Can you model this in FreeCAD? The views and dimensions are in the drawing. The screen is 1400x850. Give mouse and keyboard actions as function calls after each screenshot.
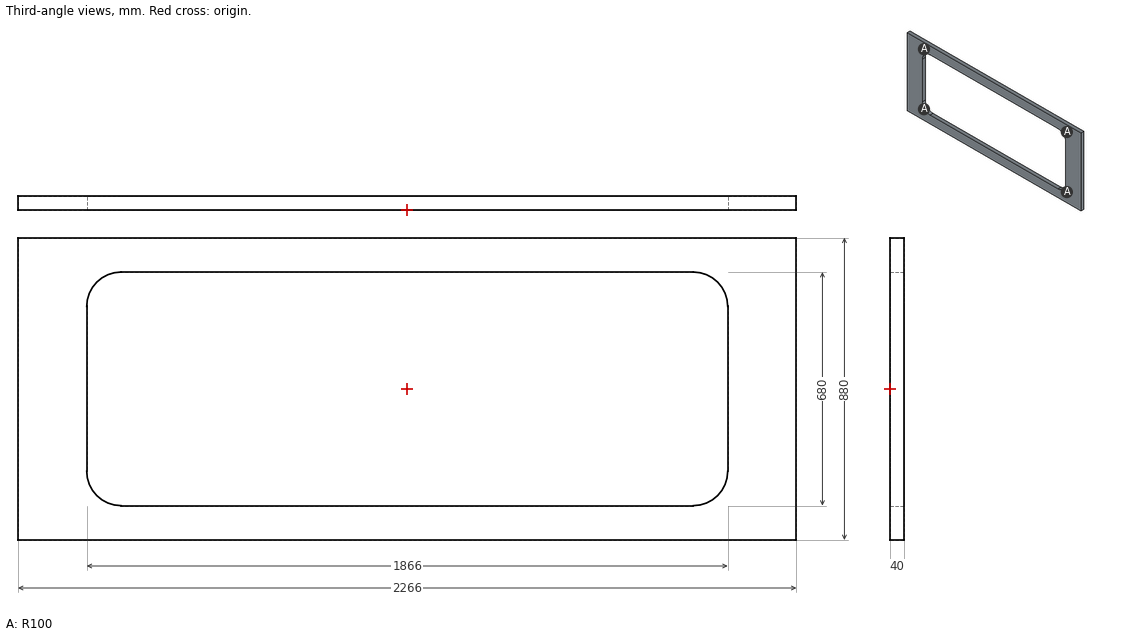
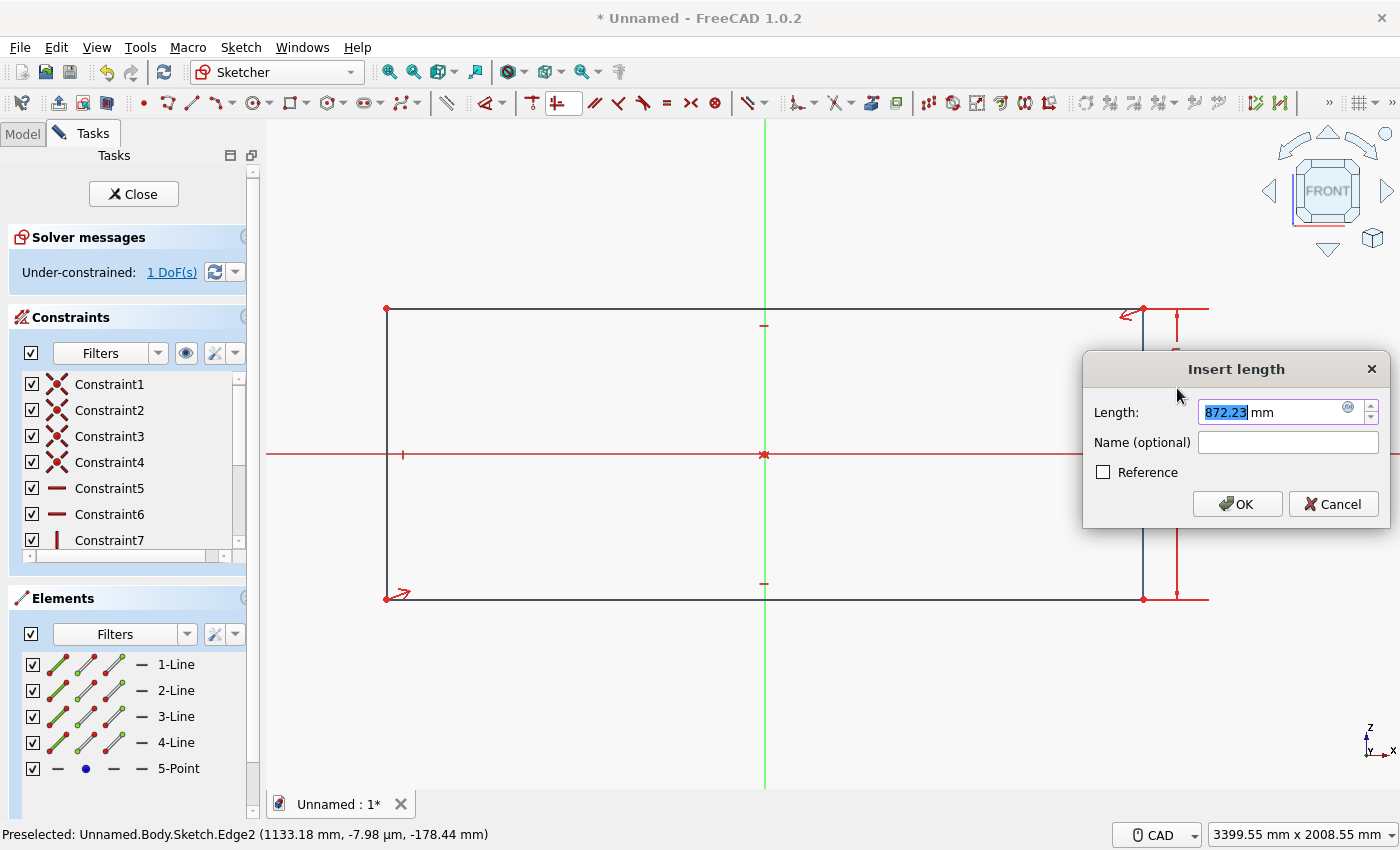
text(880)
key(Return)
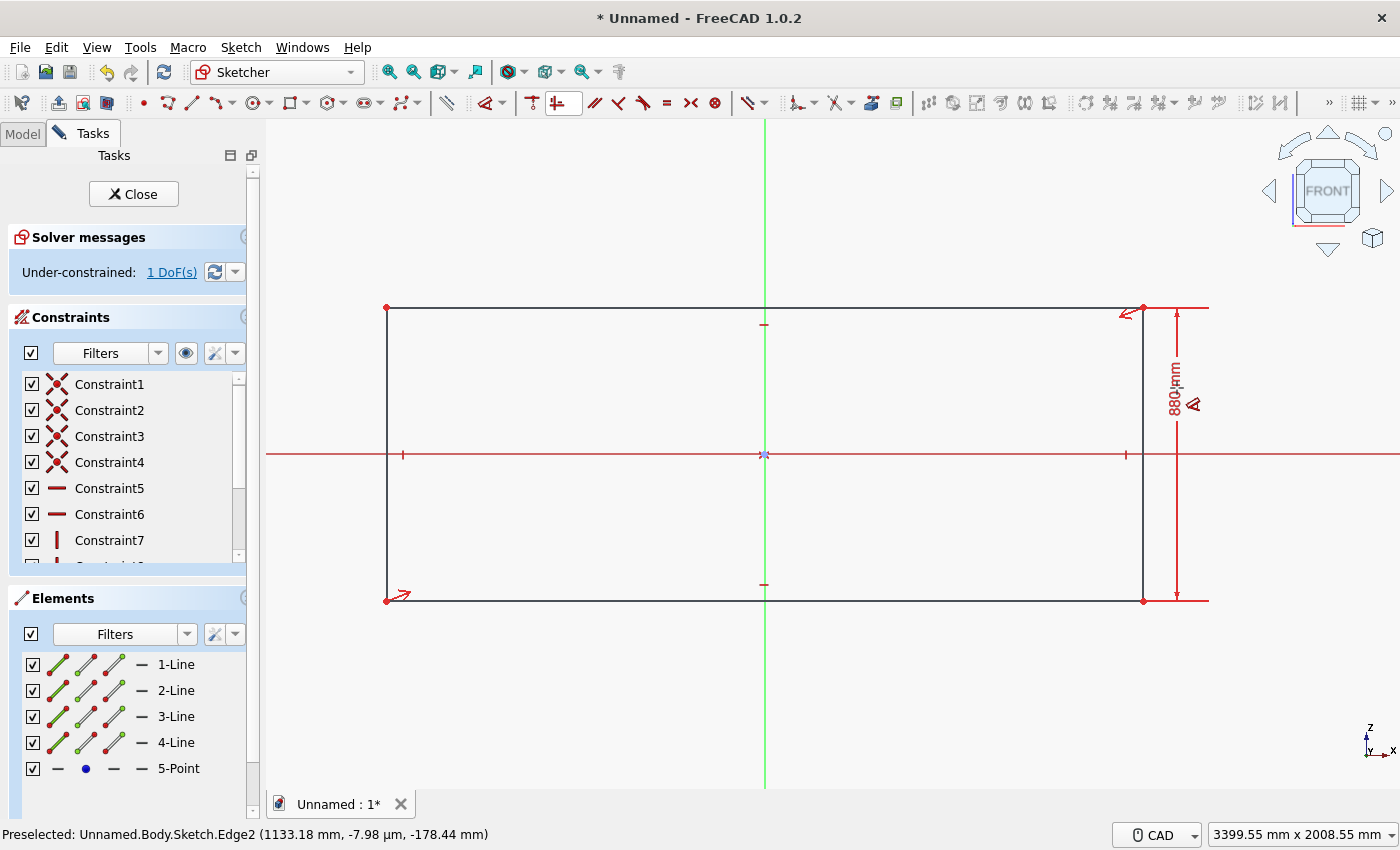
click(614, 601)
click(591, 635)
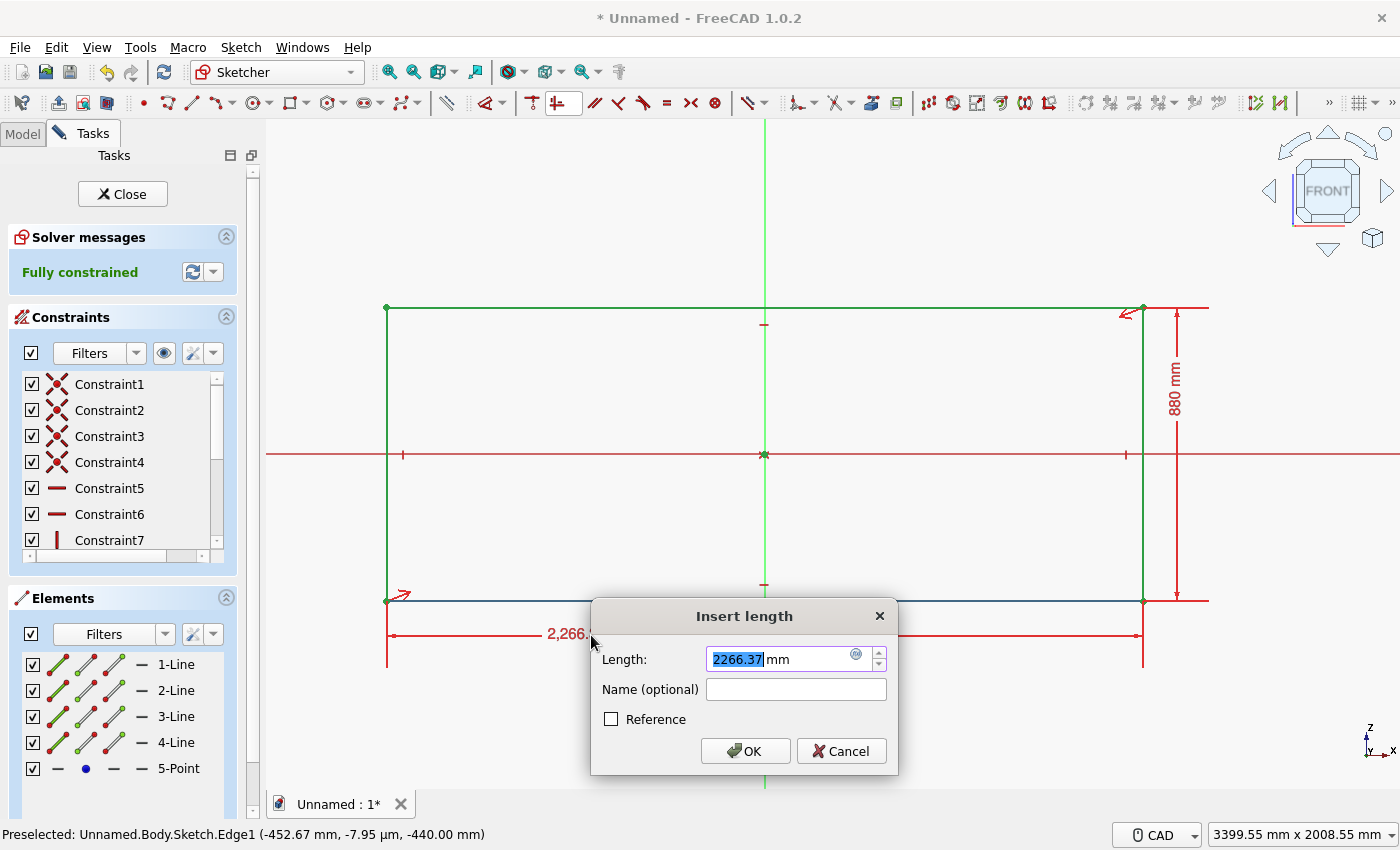
text(2266)
key(Return)
key(Escape)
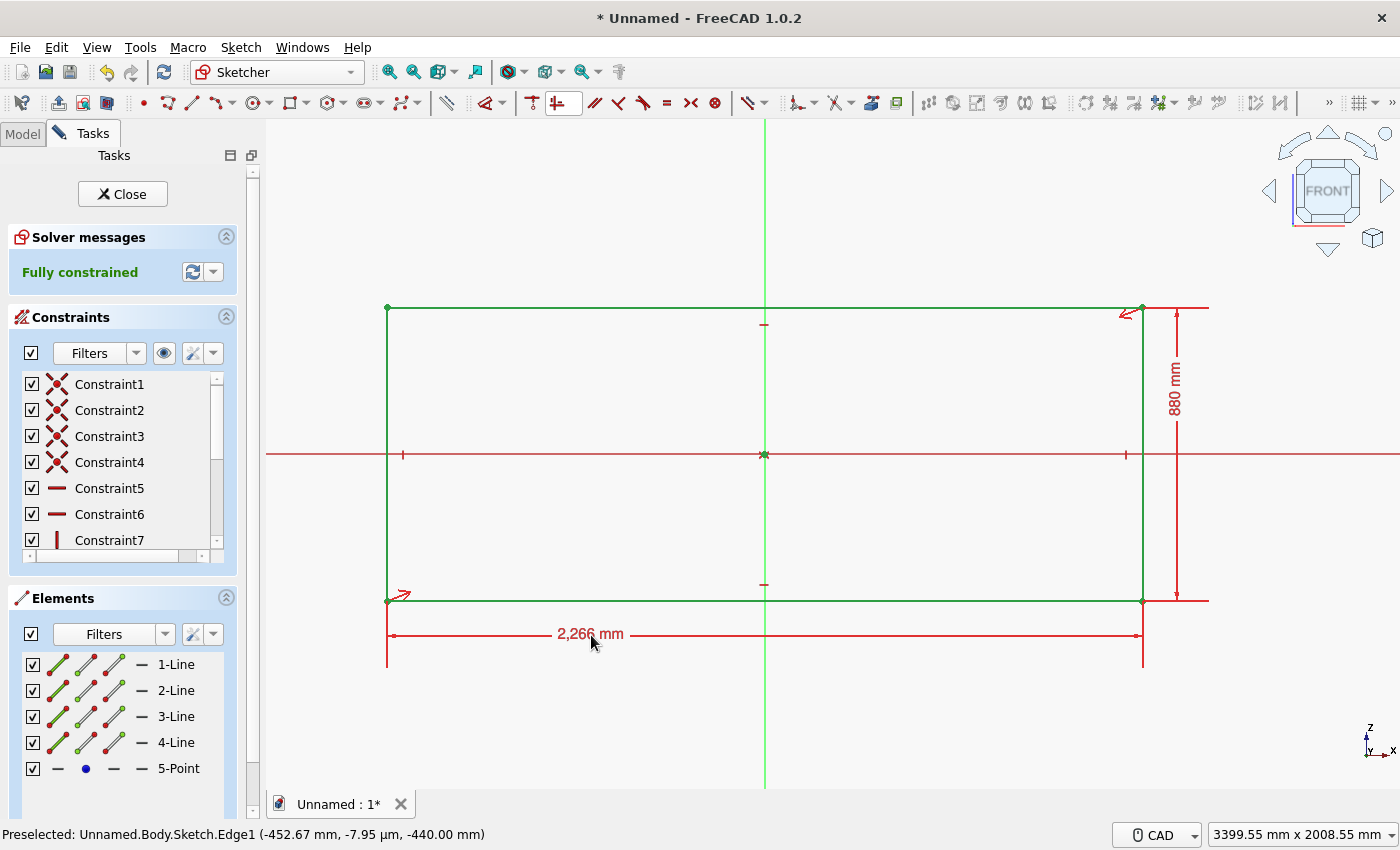
click(123, 194)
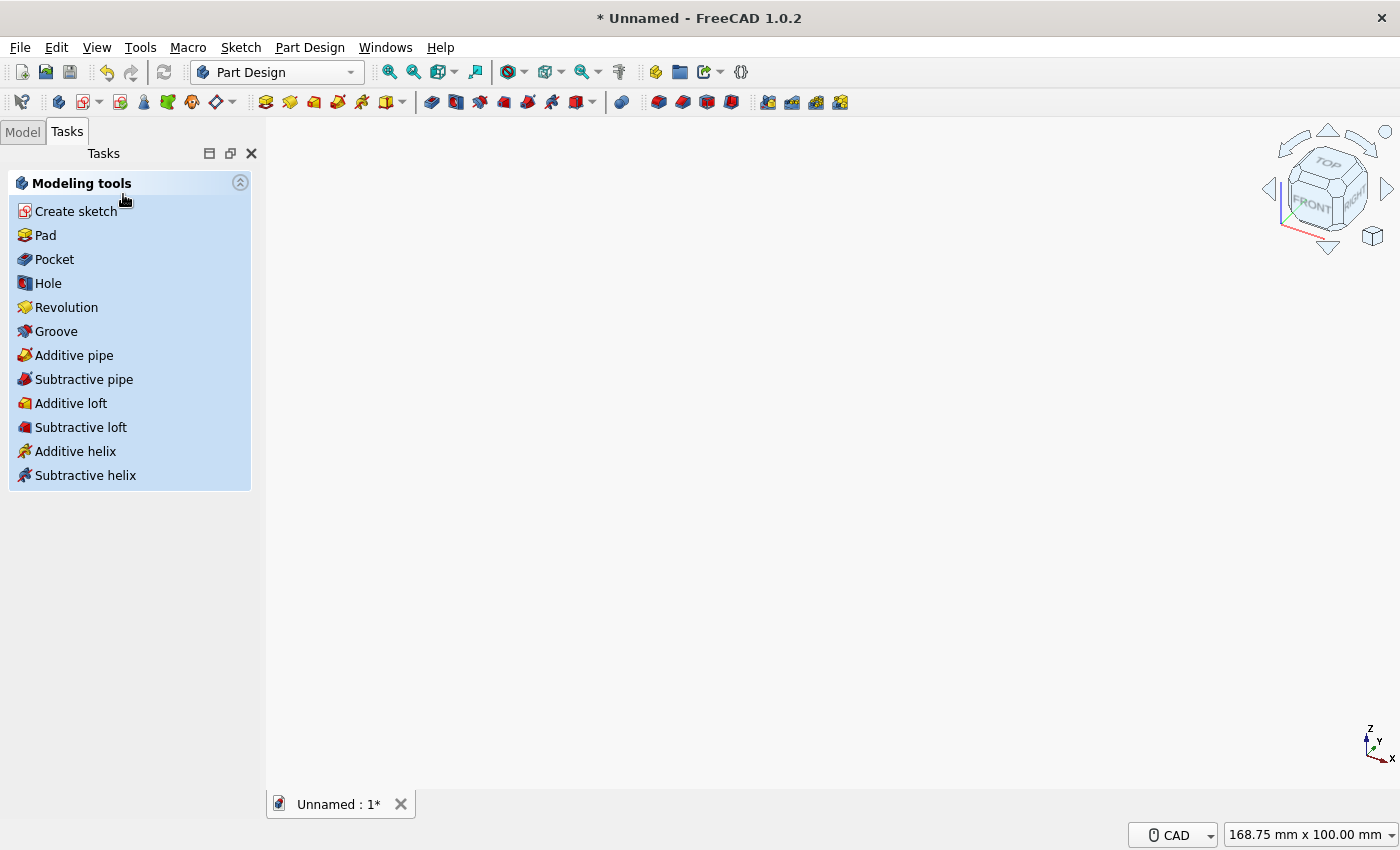
click(266, 102)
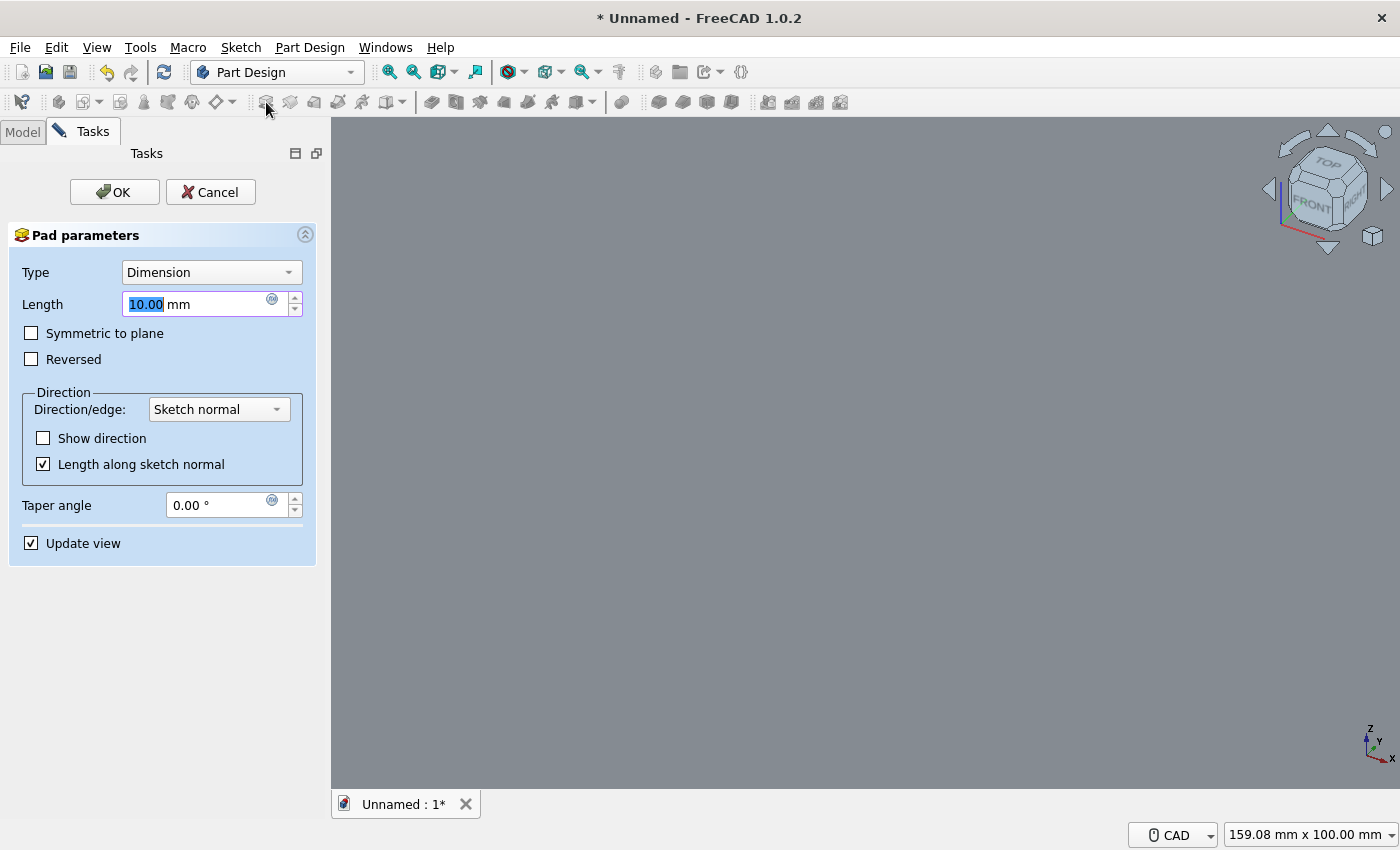
text(40)
key(Tab)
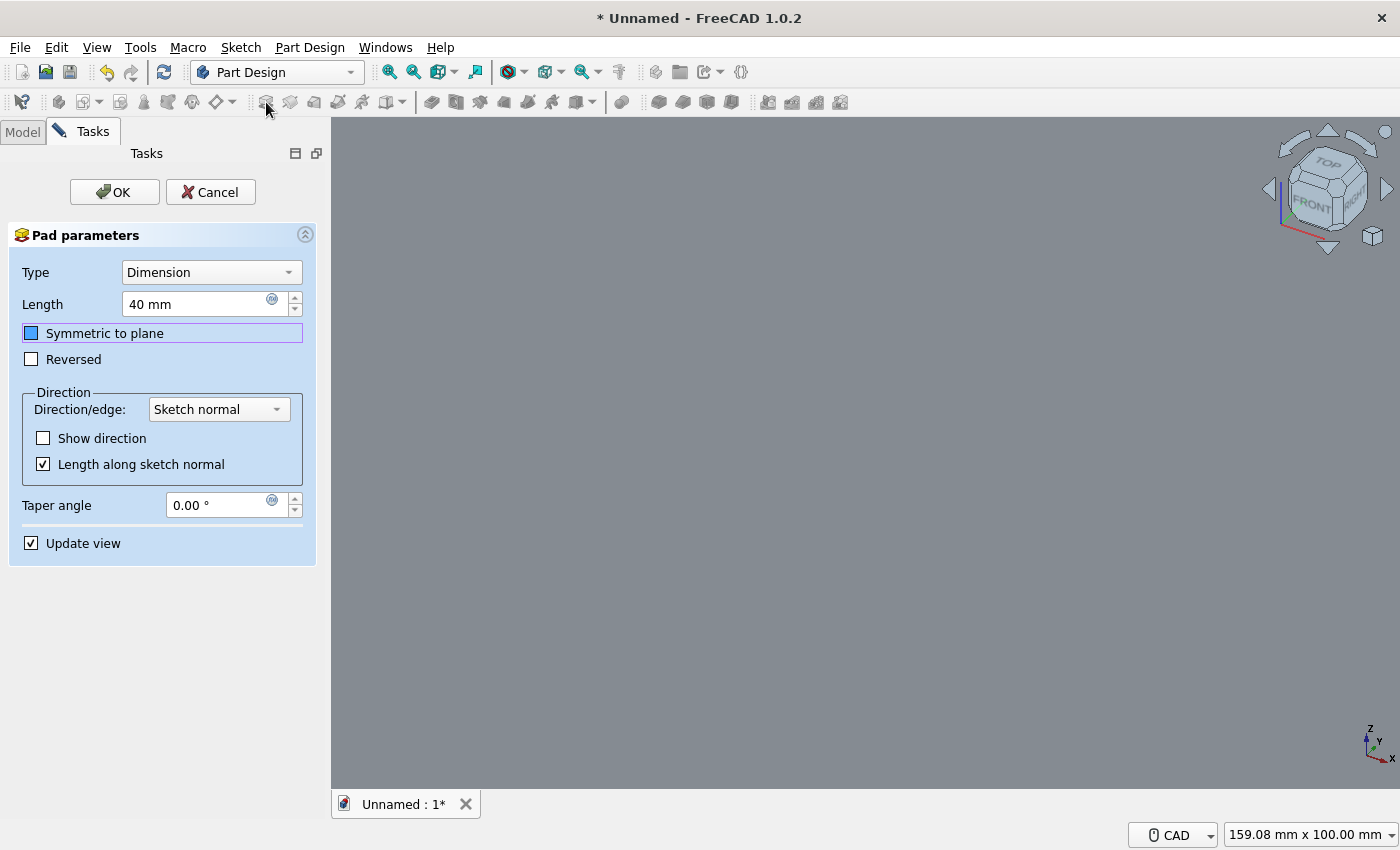
click(30, 359)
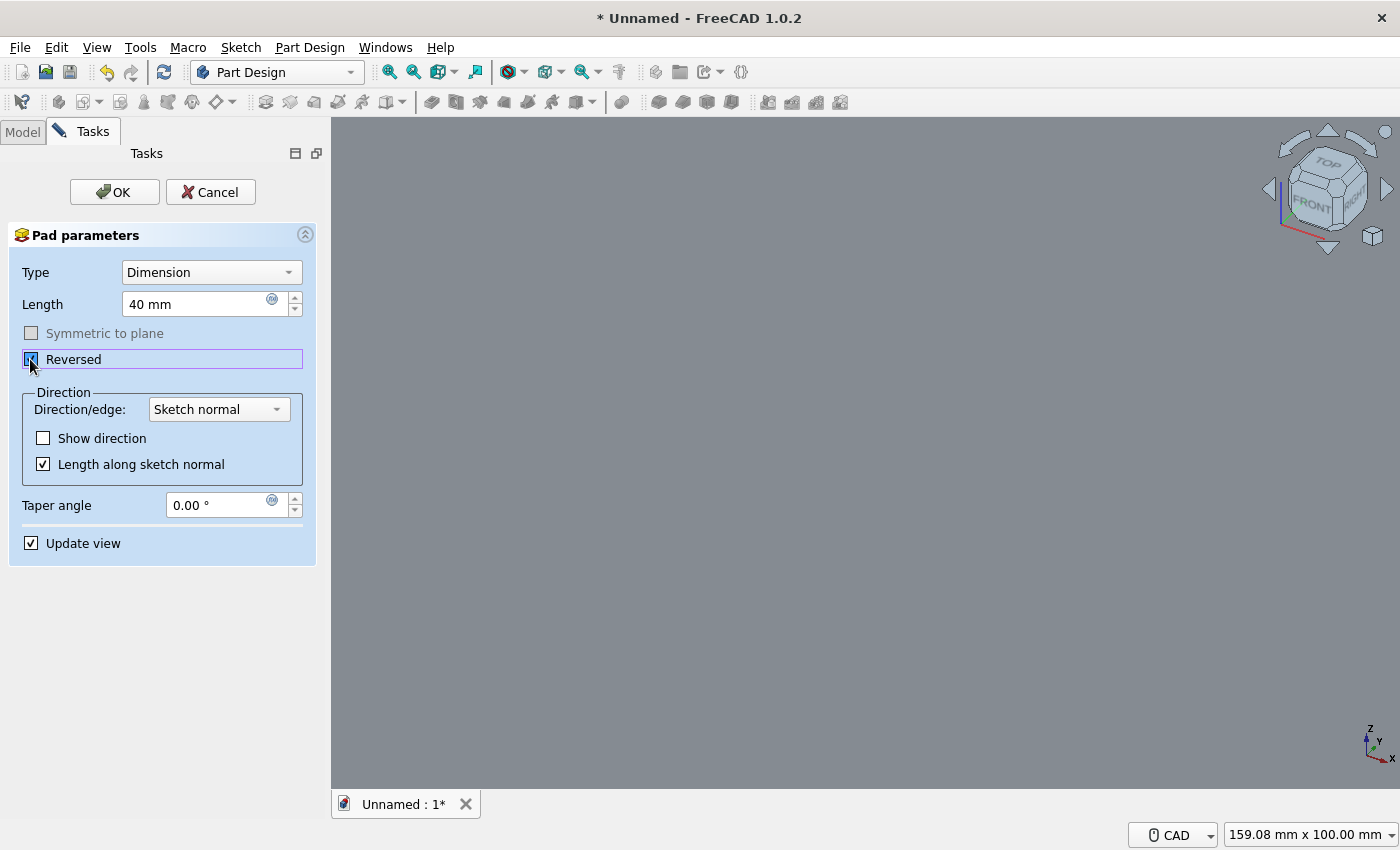
click(115, 192)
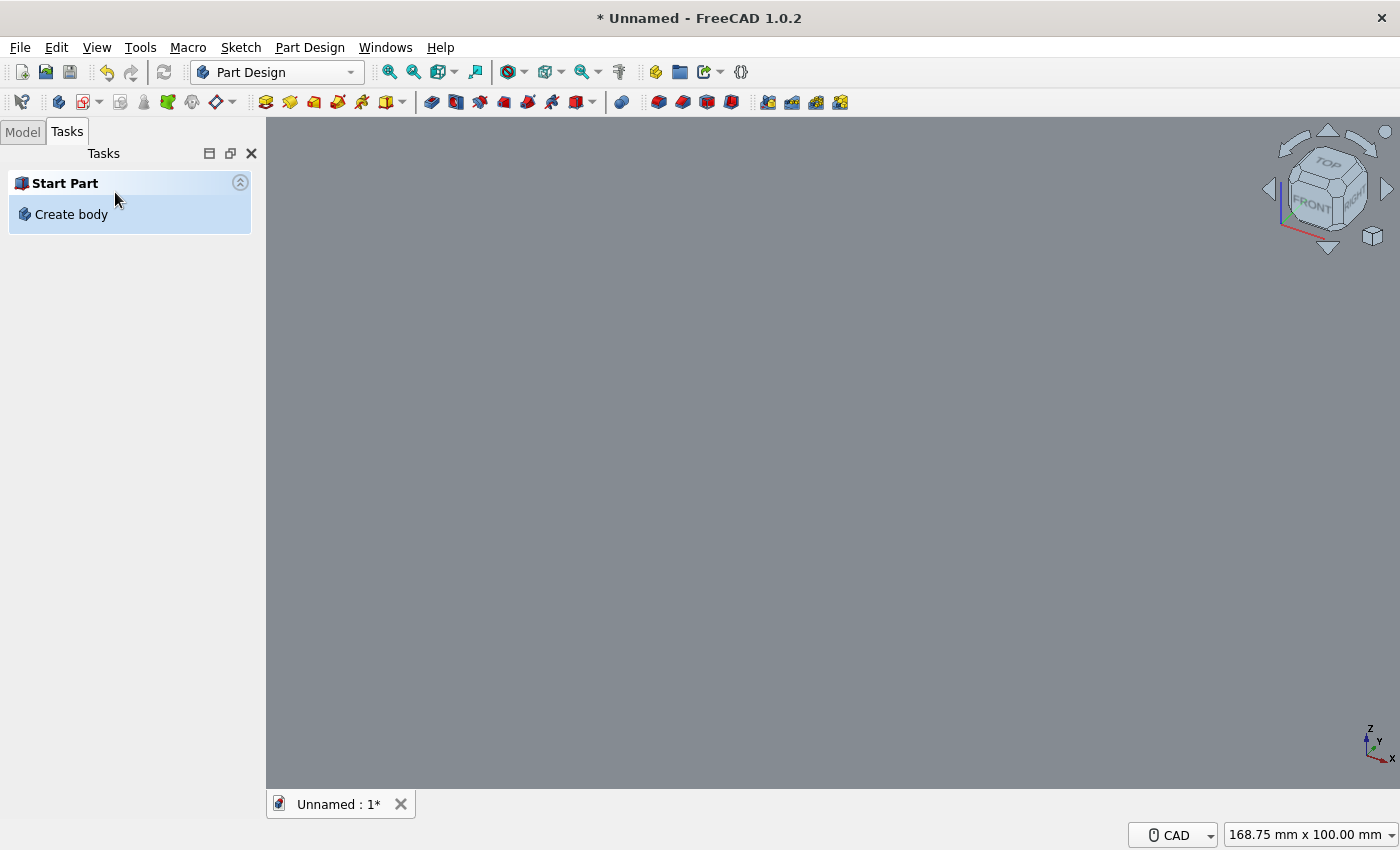
key(v)
key(f)